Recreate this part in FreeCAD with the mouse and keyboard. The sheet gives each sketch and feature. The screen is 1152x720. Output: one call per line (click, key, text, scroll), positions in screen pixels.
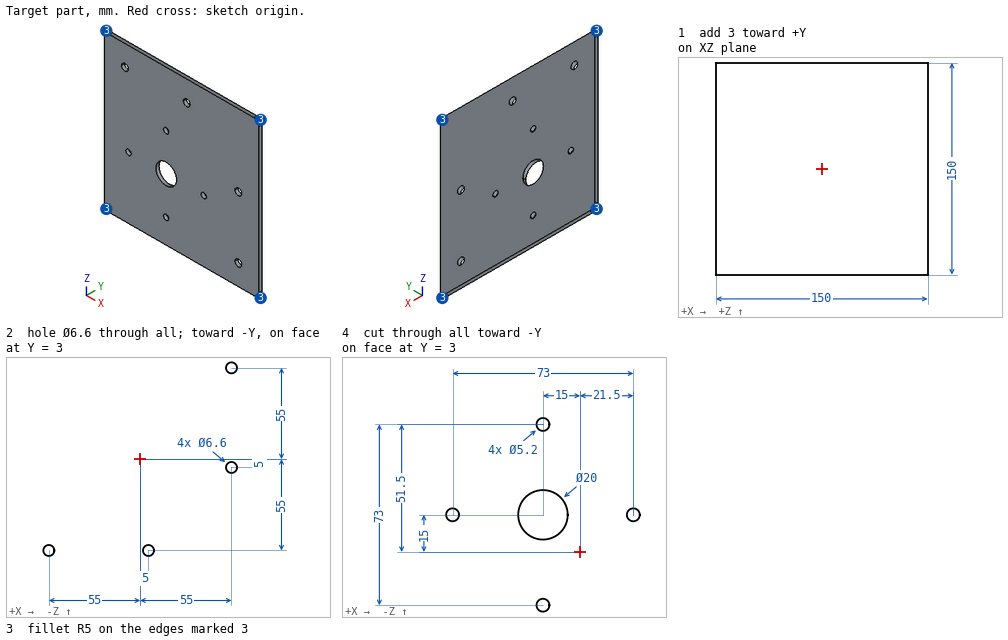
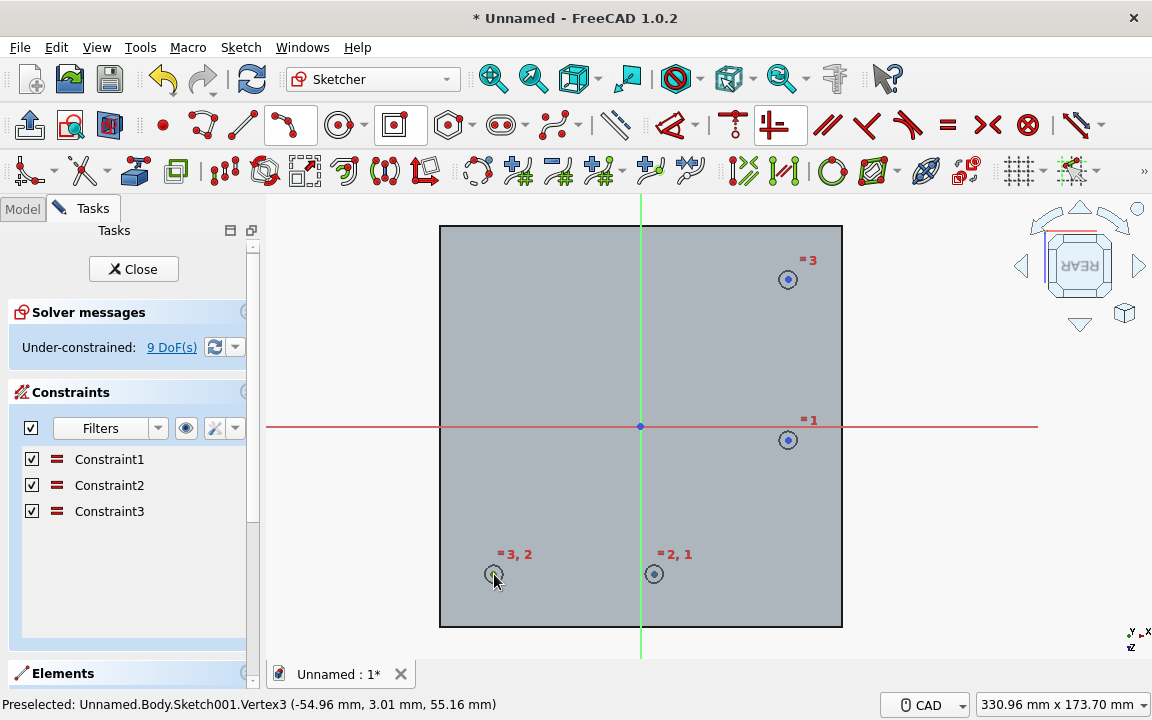
key(h)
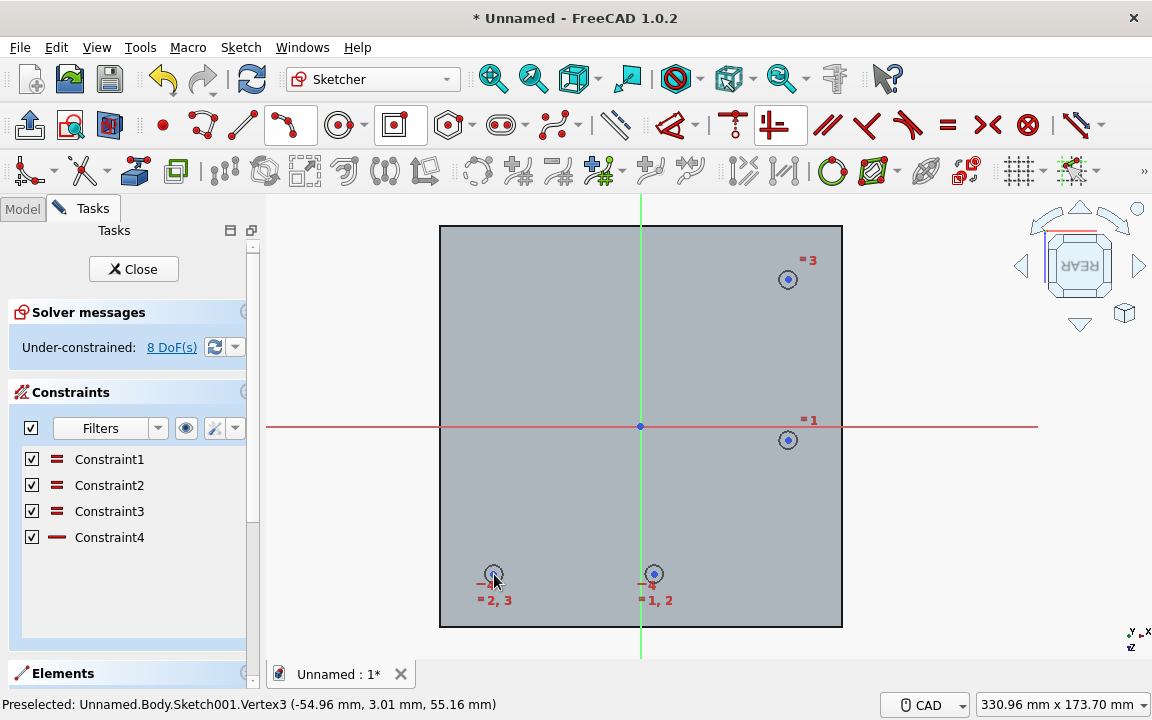
click(788, 440)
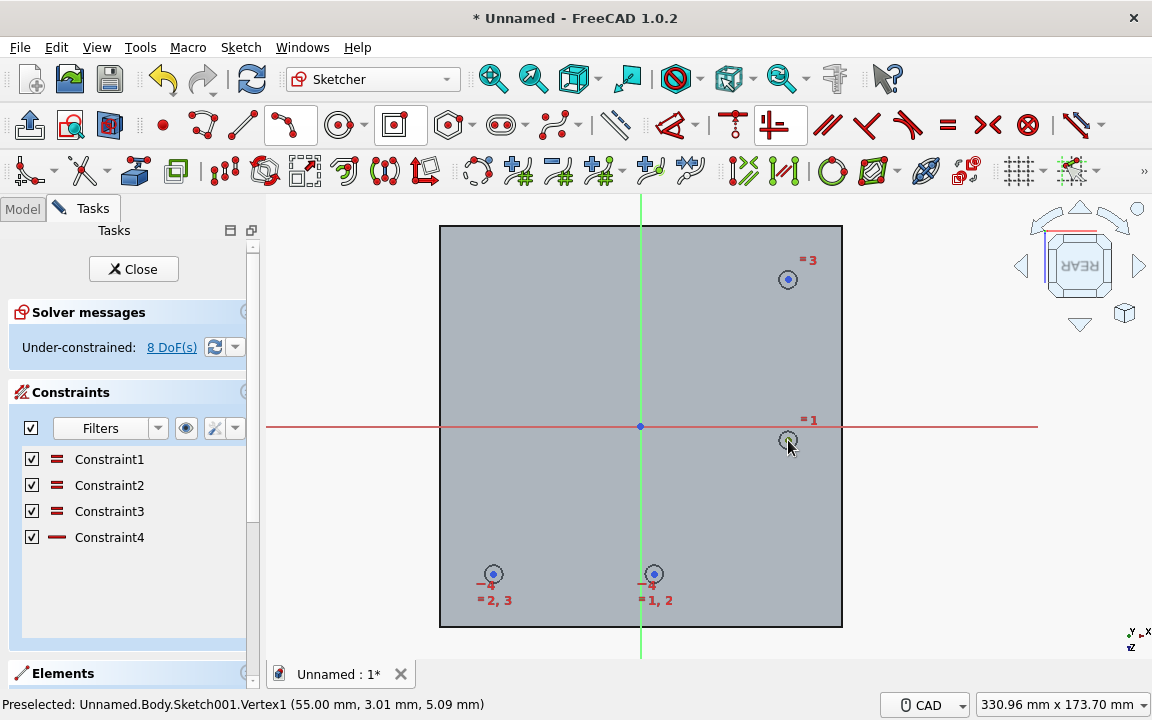
click(788, 280)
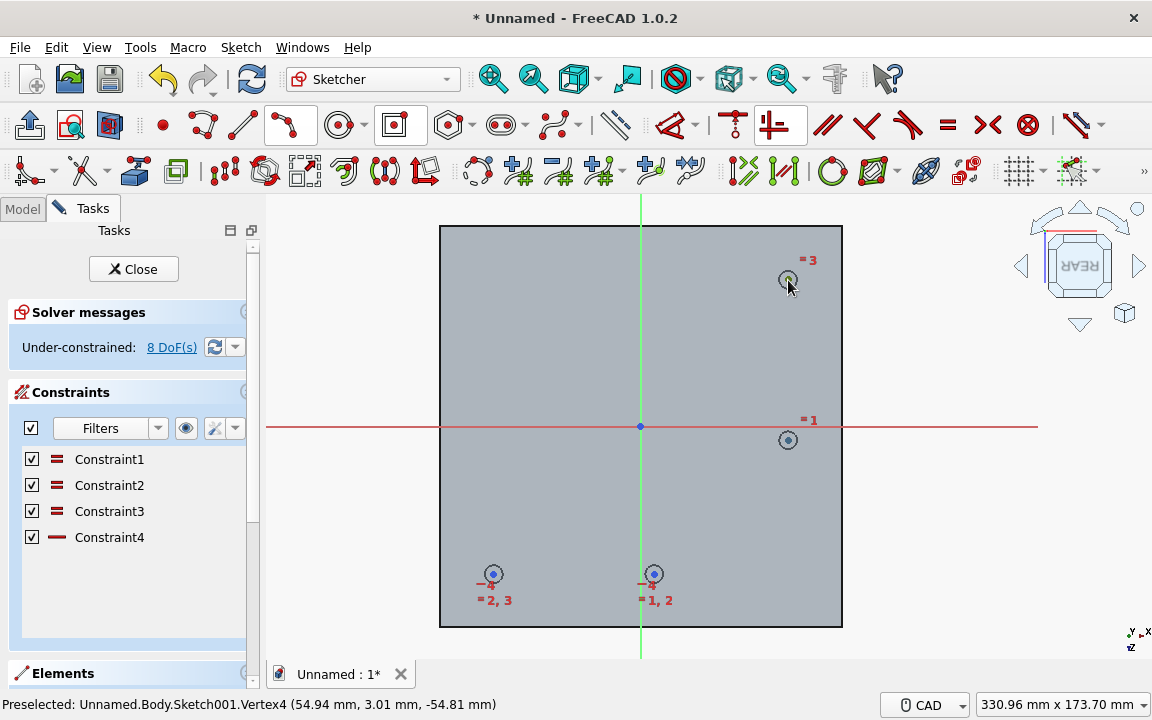
click(802, 126)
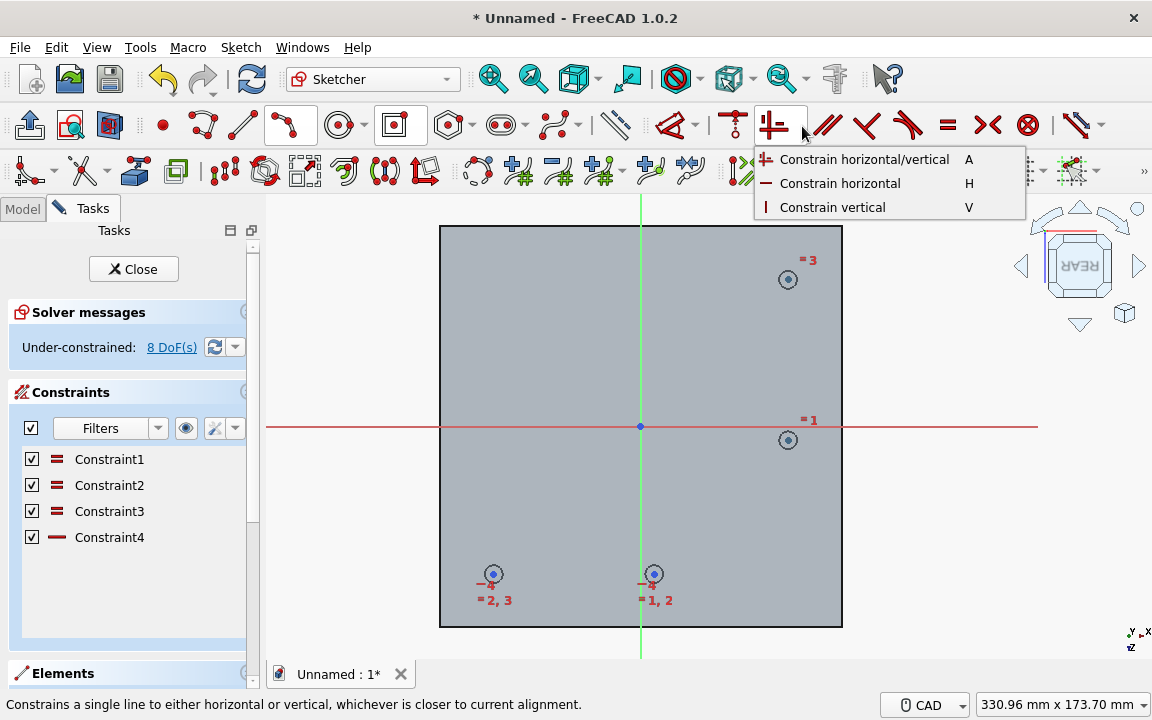
click(890, 207)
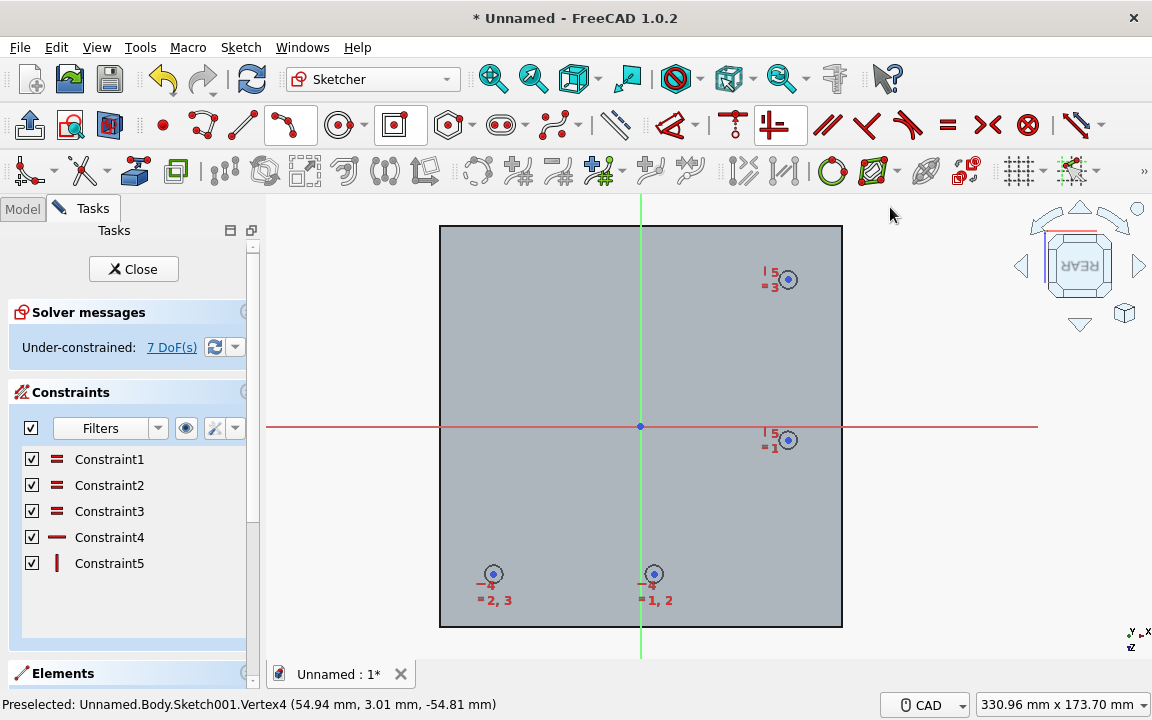
click(670, 126)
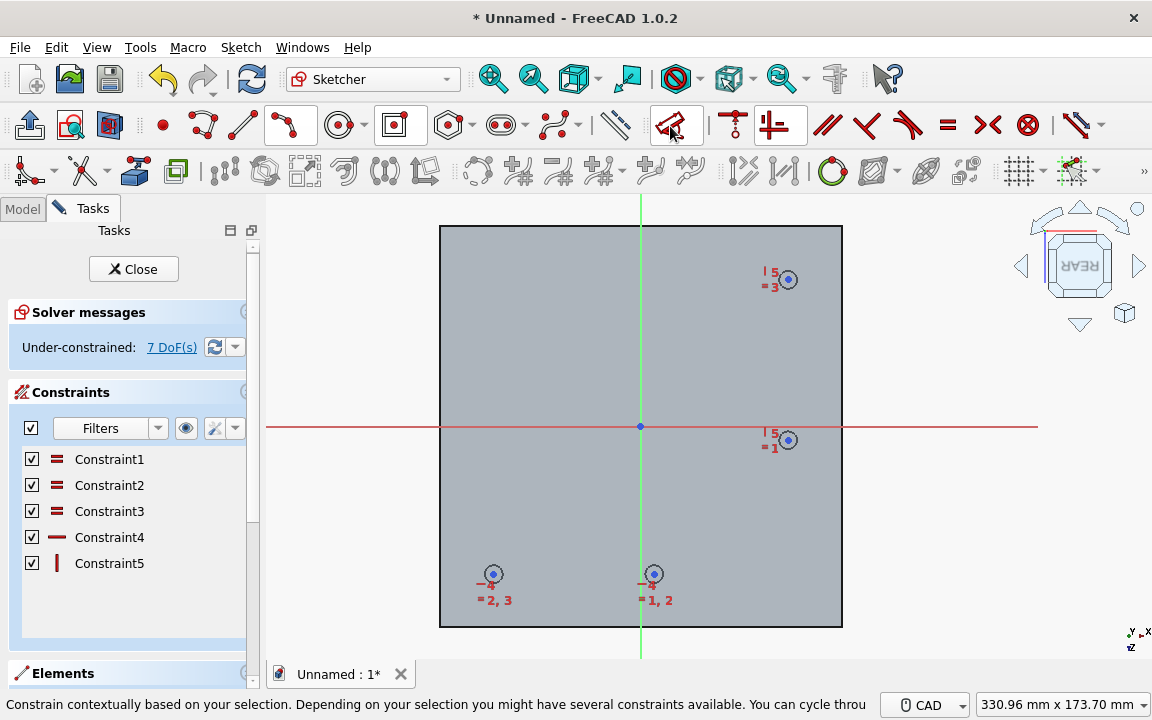
scroll(788, 449, up, 5)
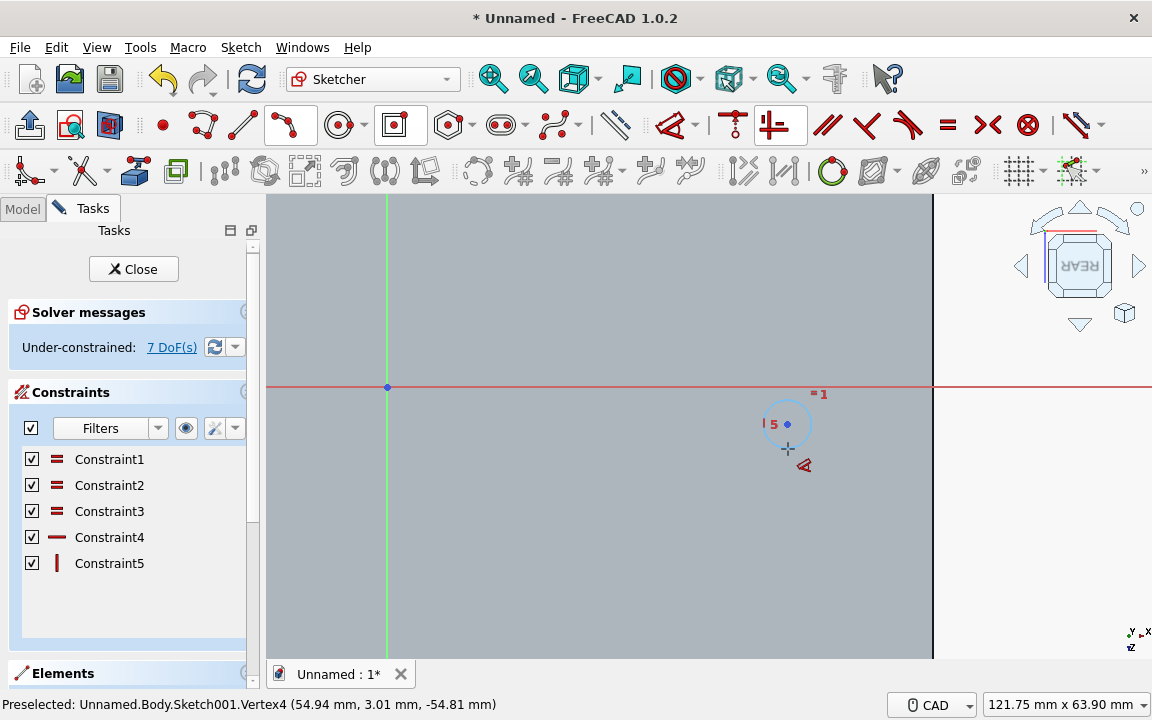
click(787, 448)
click(786, 480)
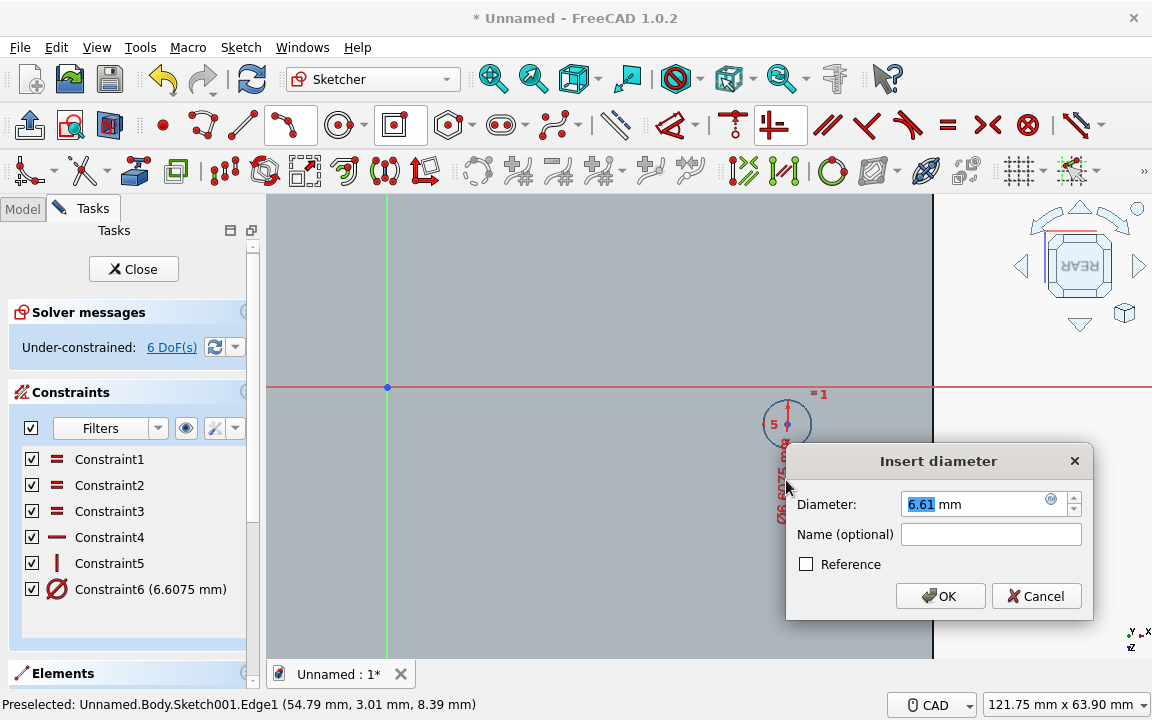
text(6.6)
key(Return)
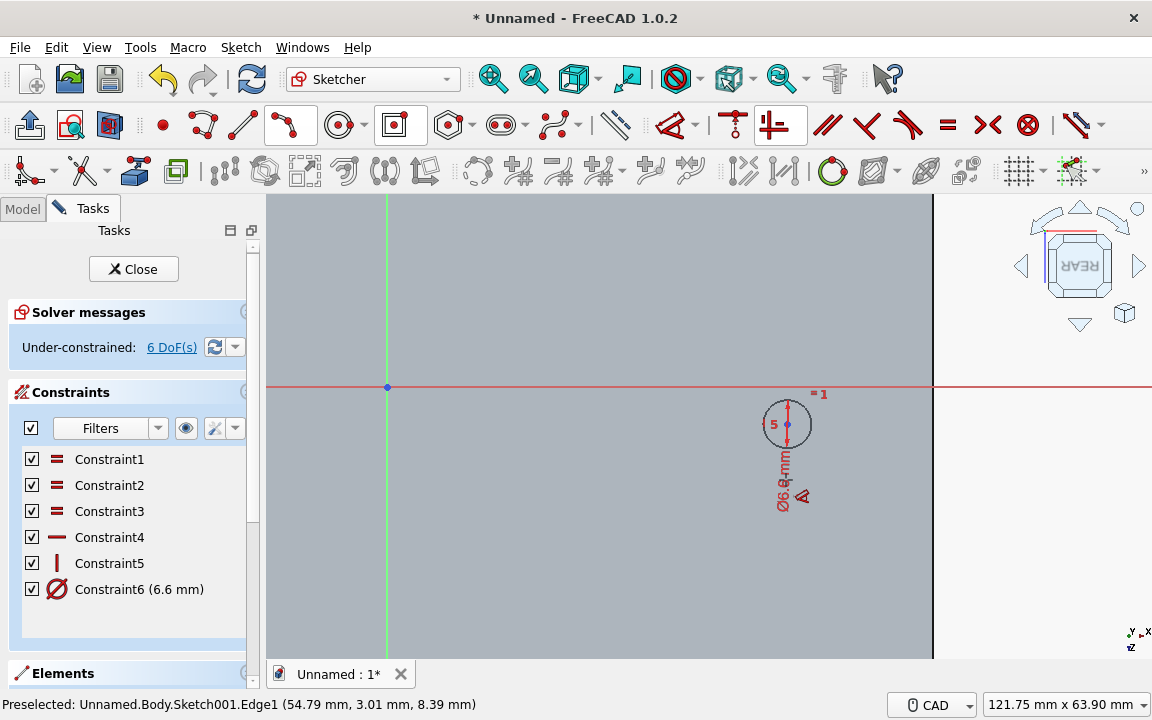
click(787, 424)
click(821, 406)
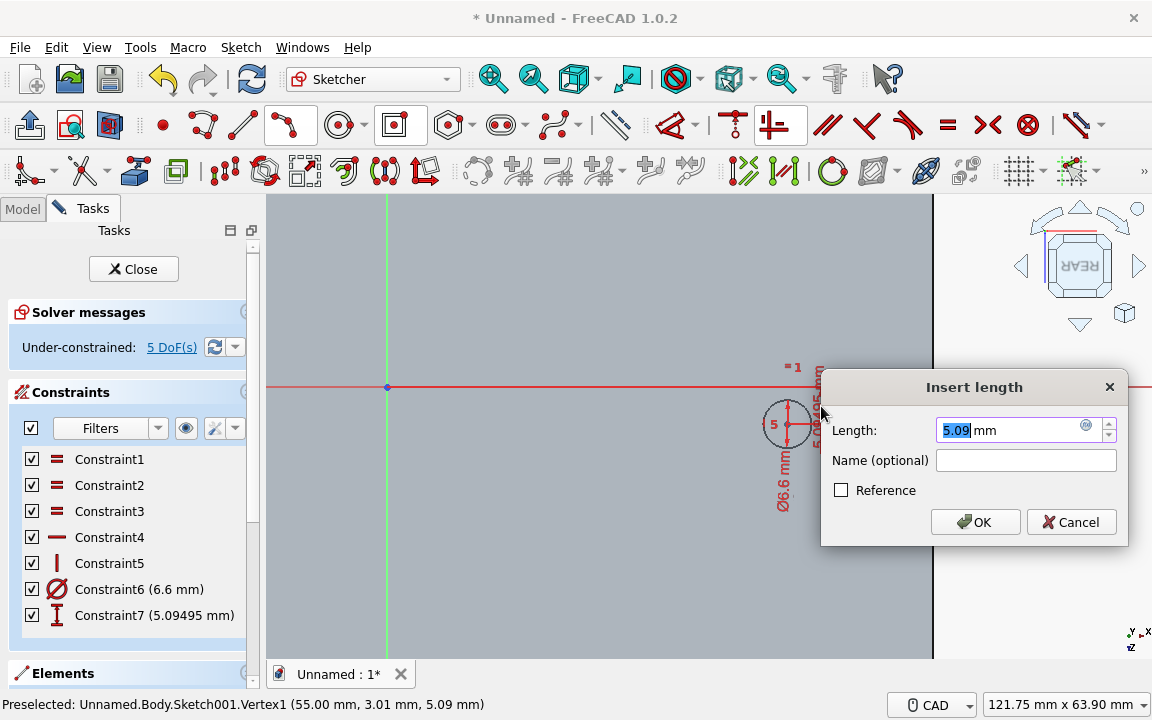
text(5)
key(Return)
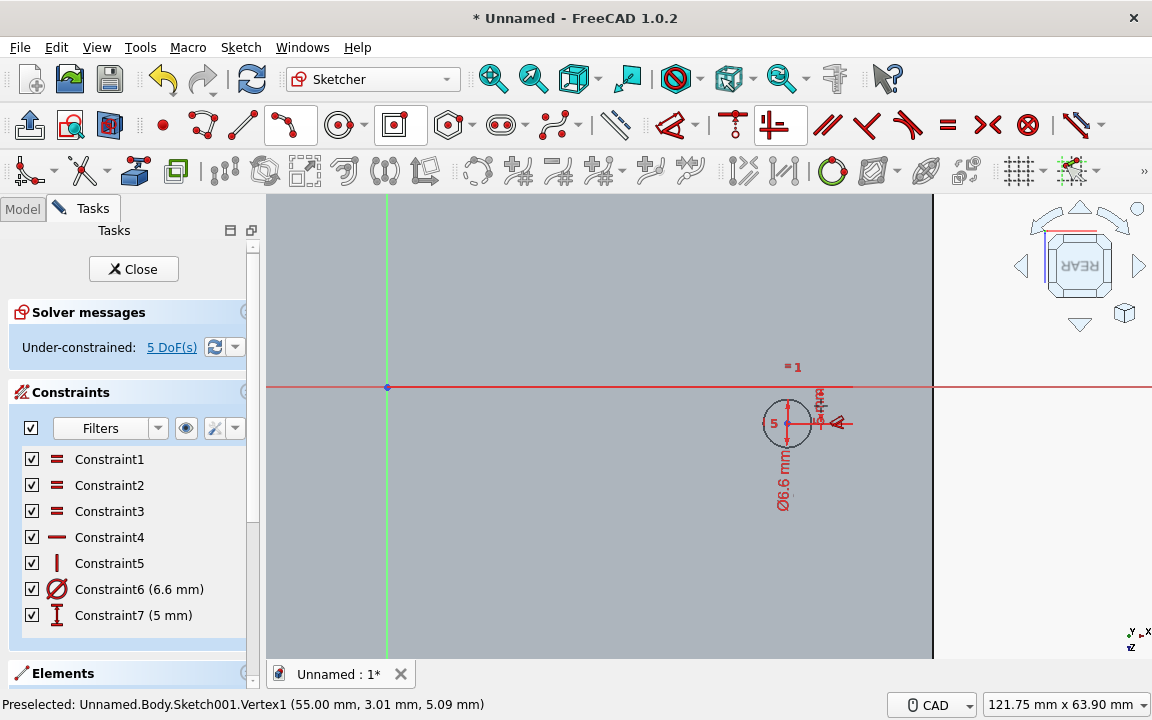
scroll(788, 449, down, 5)